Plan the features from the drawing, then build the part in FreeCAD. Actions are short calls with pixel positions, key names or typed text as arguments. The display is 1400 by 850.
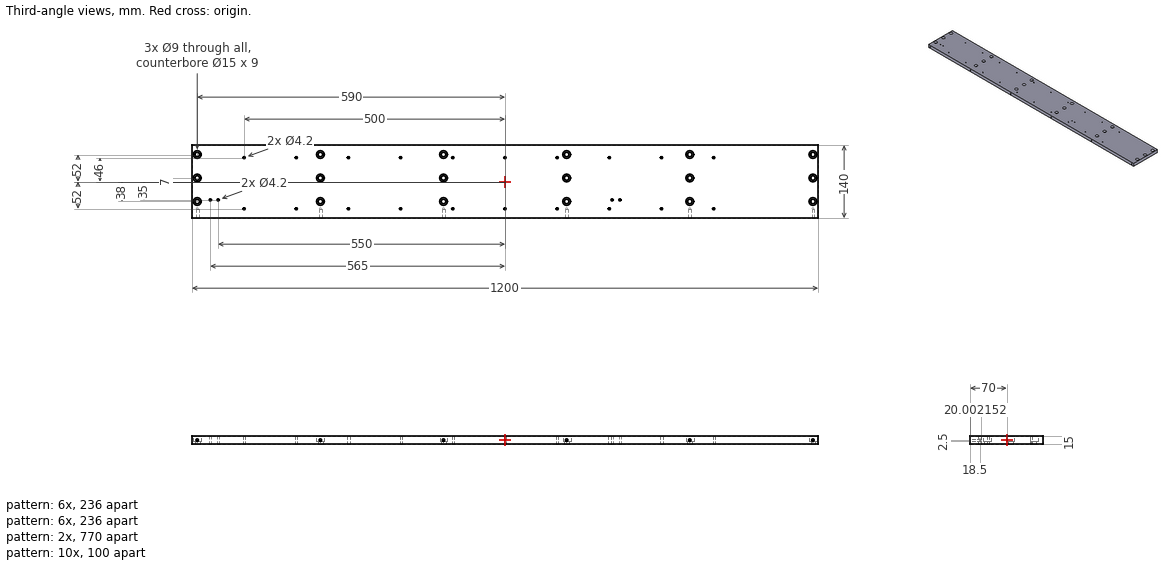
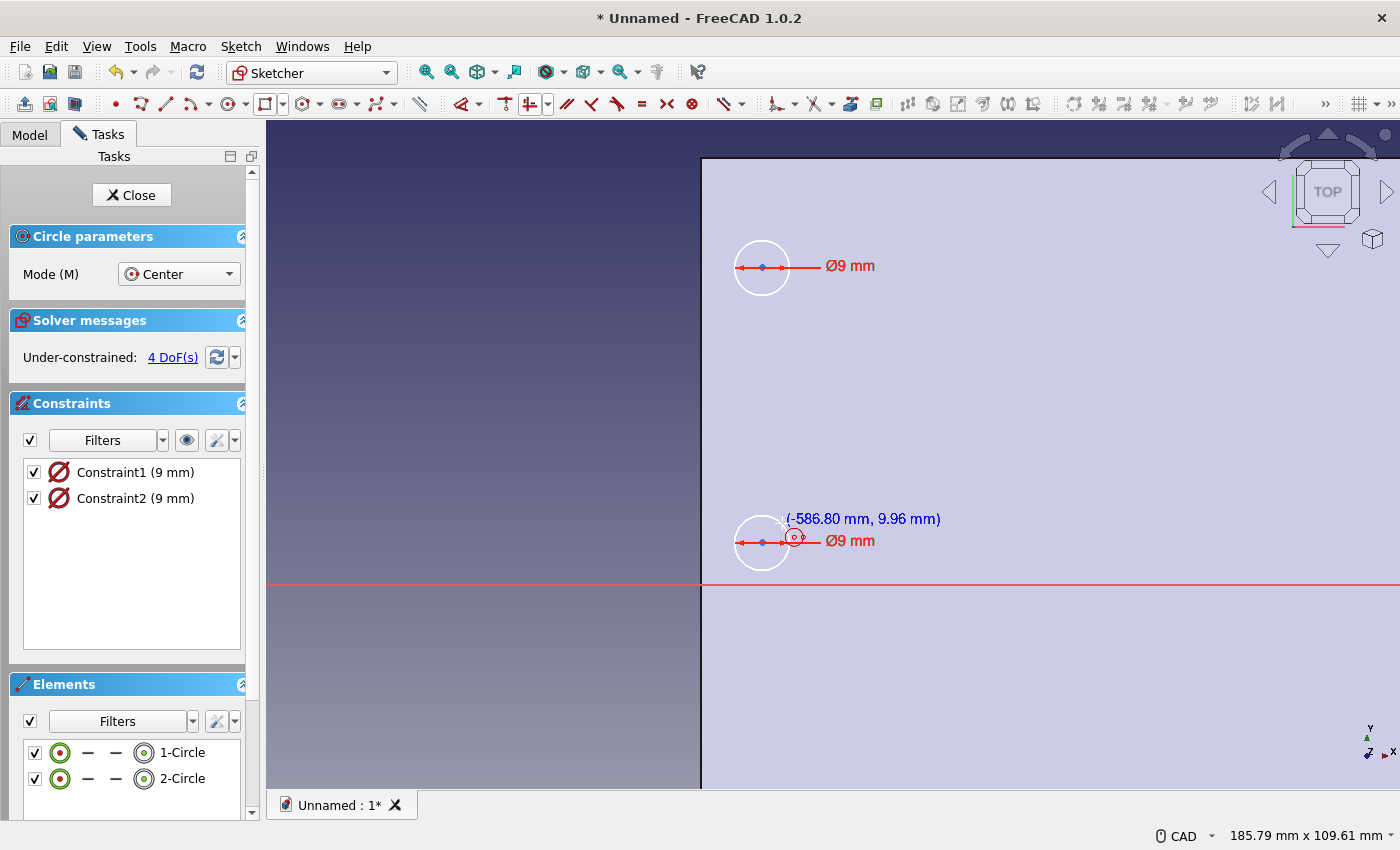
scroll(769, 276, down, 2)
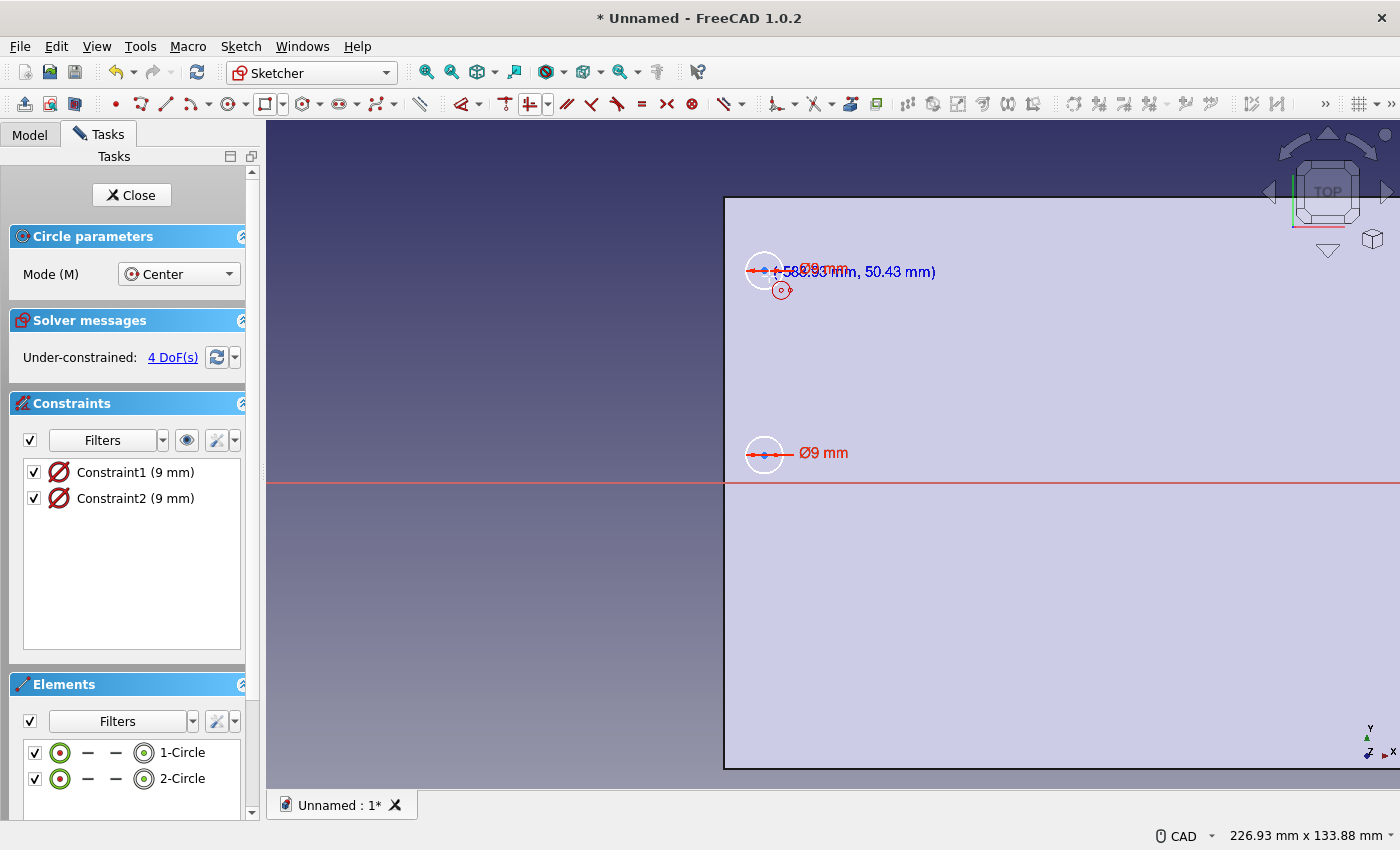
scroll(765, 639, up, 2)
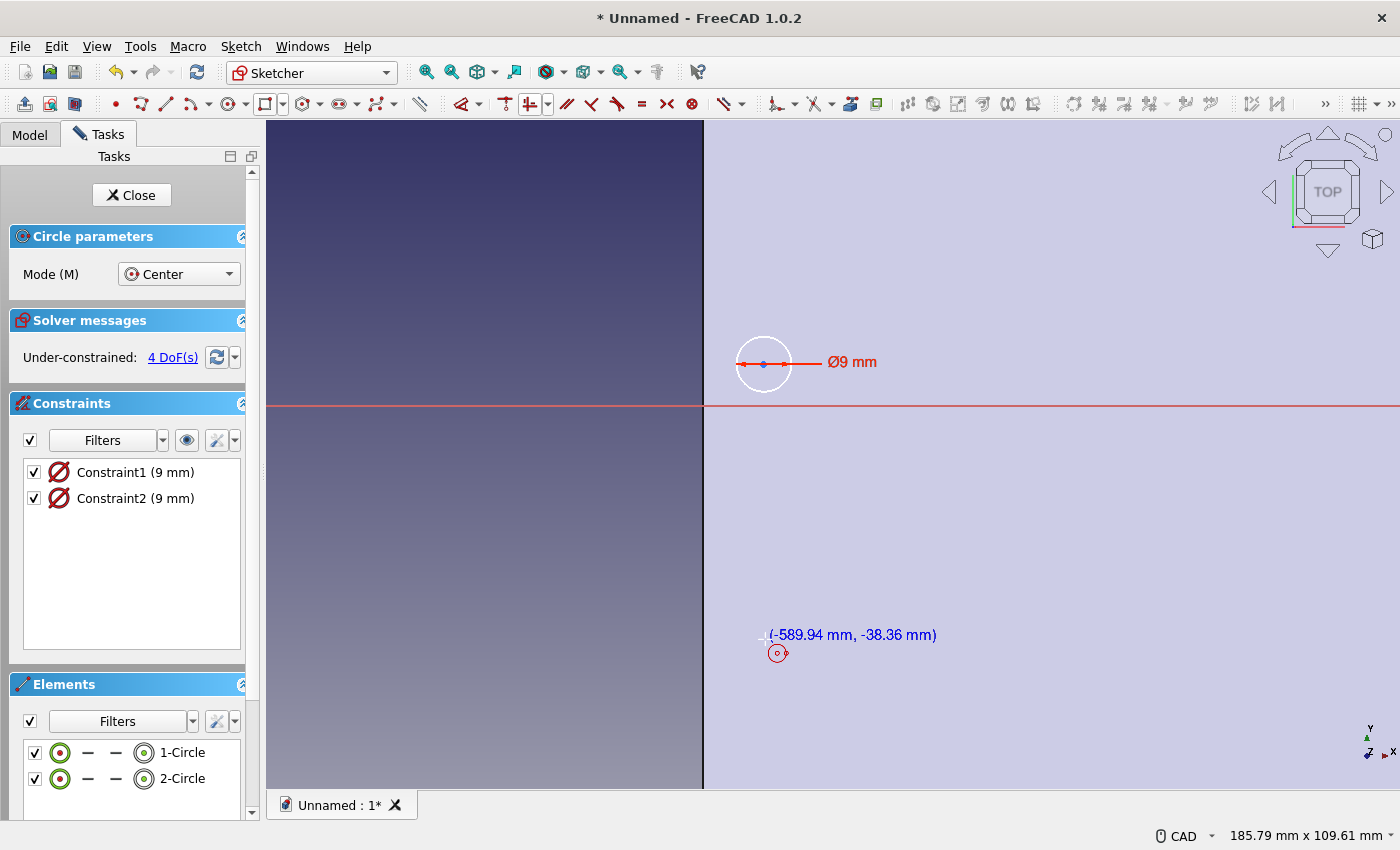
click(764, 638)
move(784, 619)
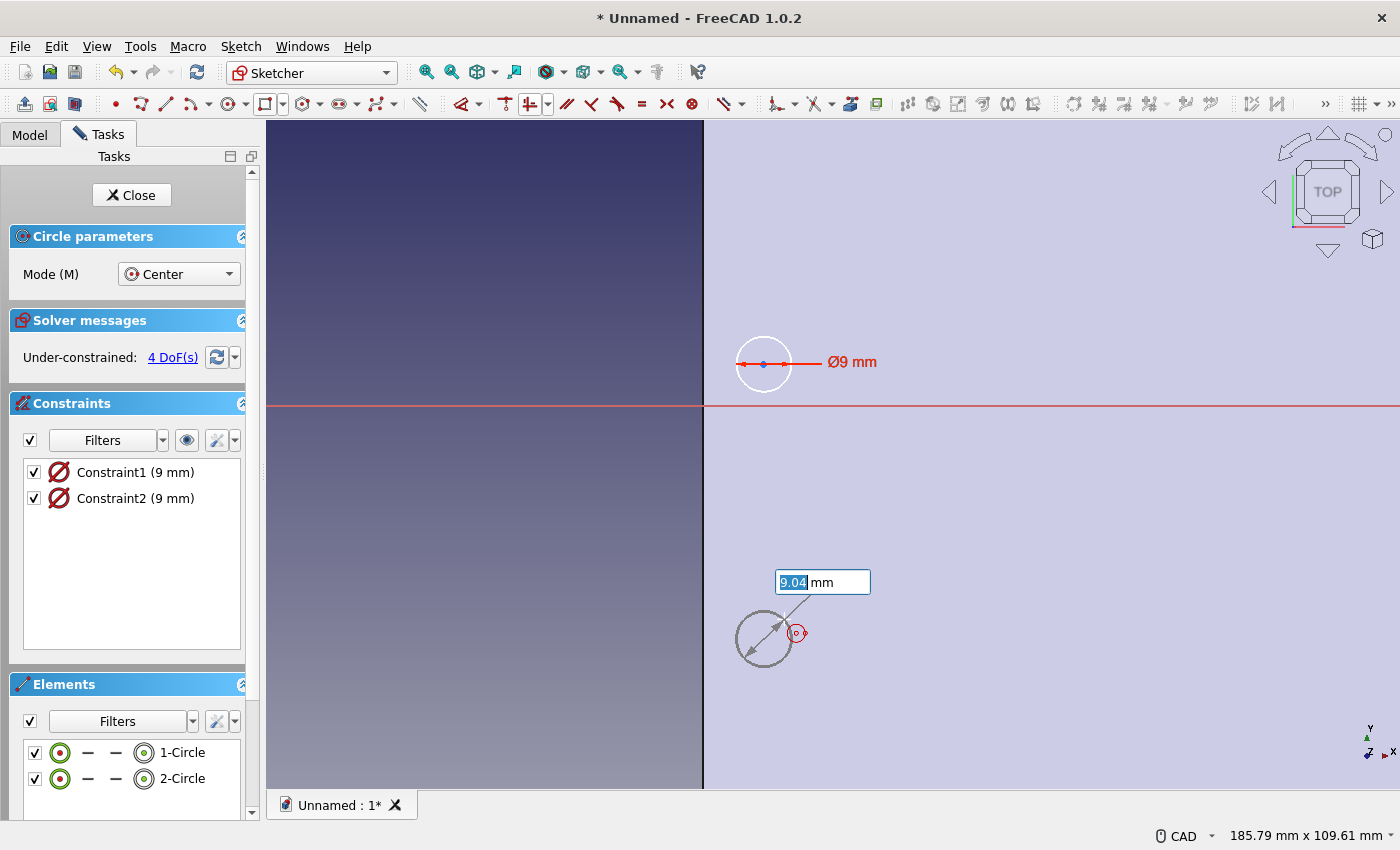
text(9)
key(Return)
key(Escape)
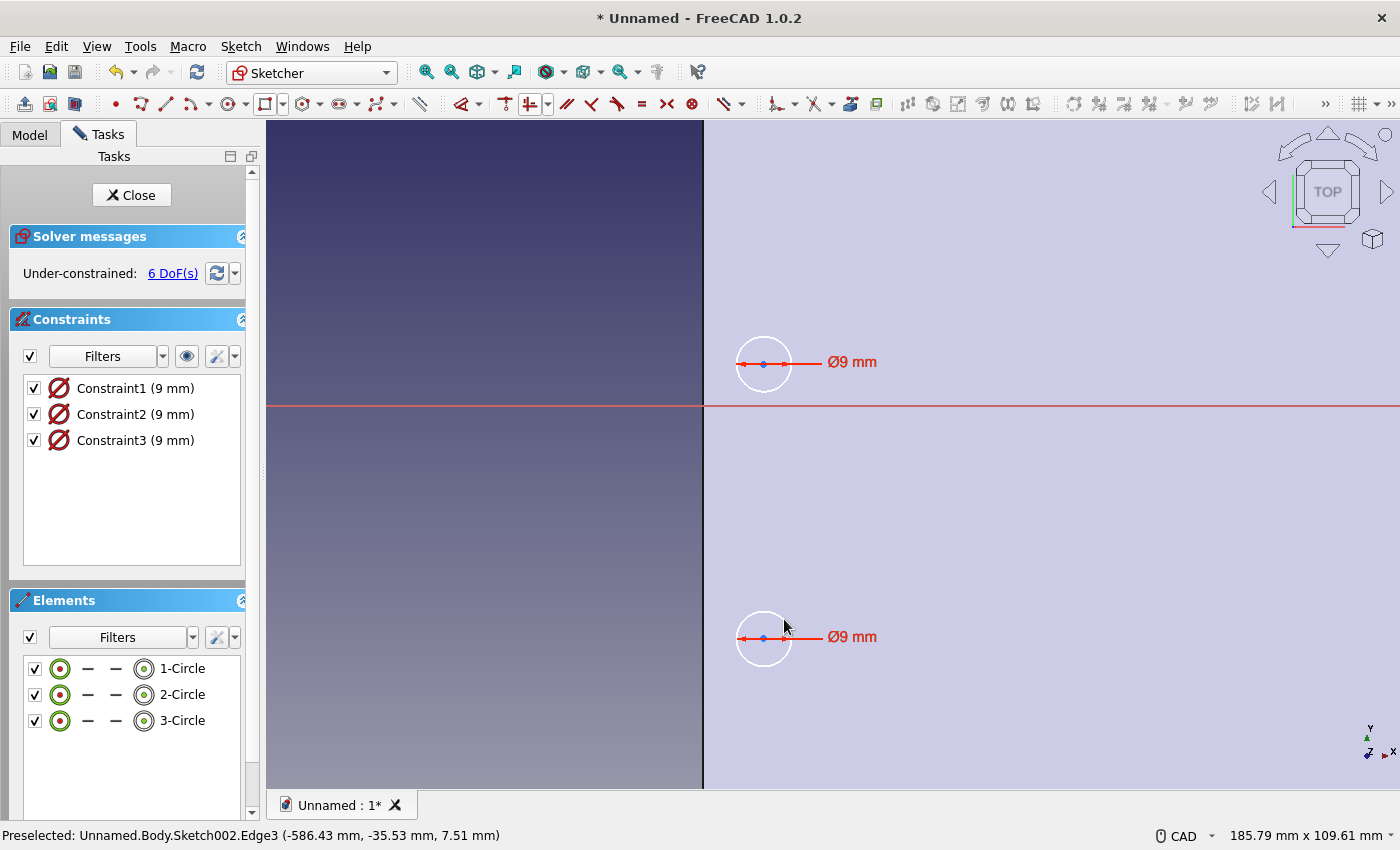
scroll(765, 640, down, 2)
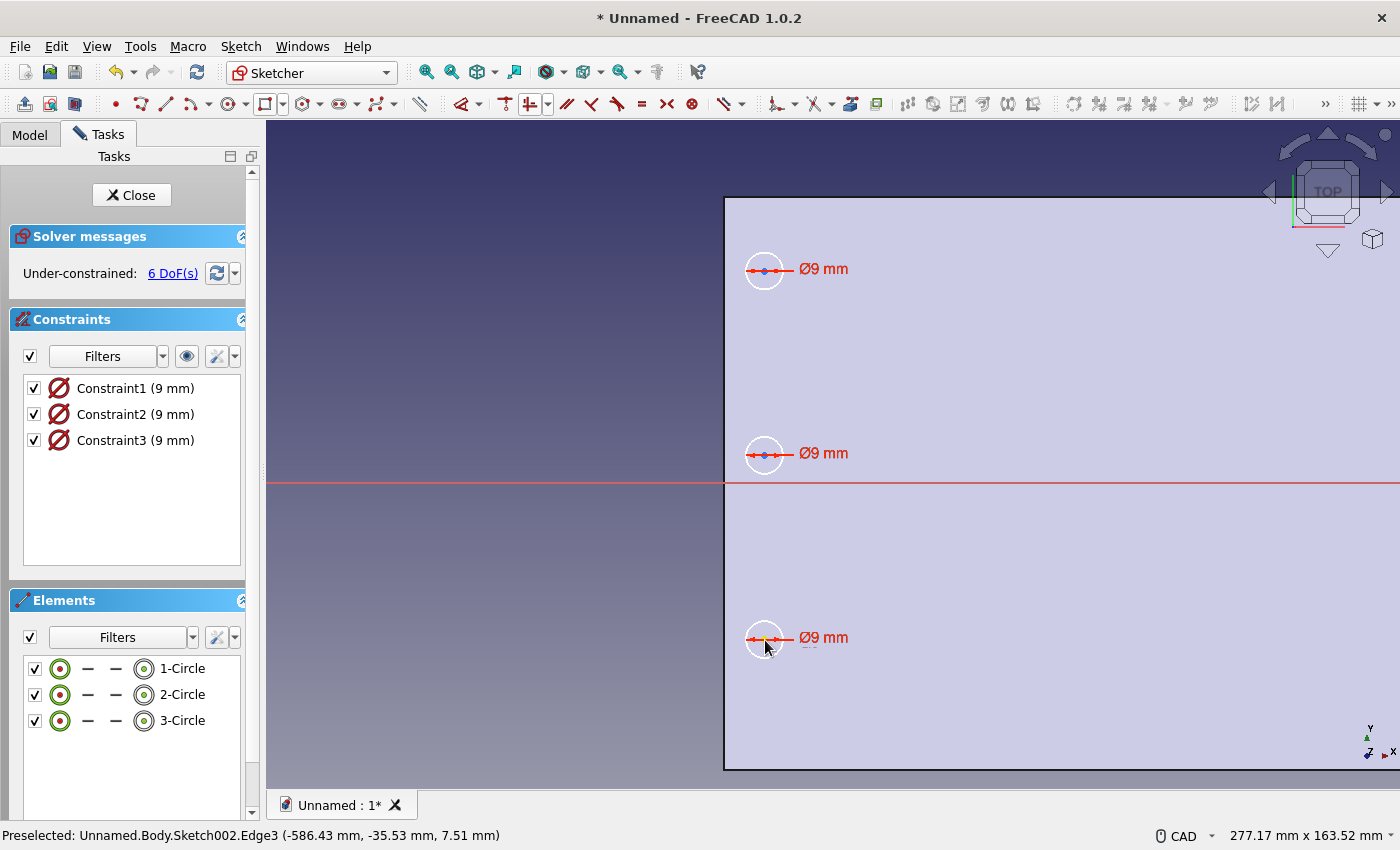
click(764, 271)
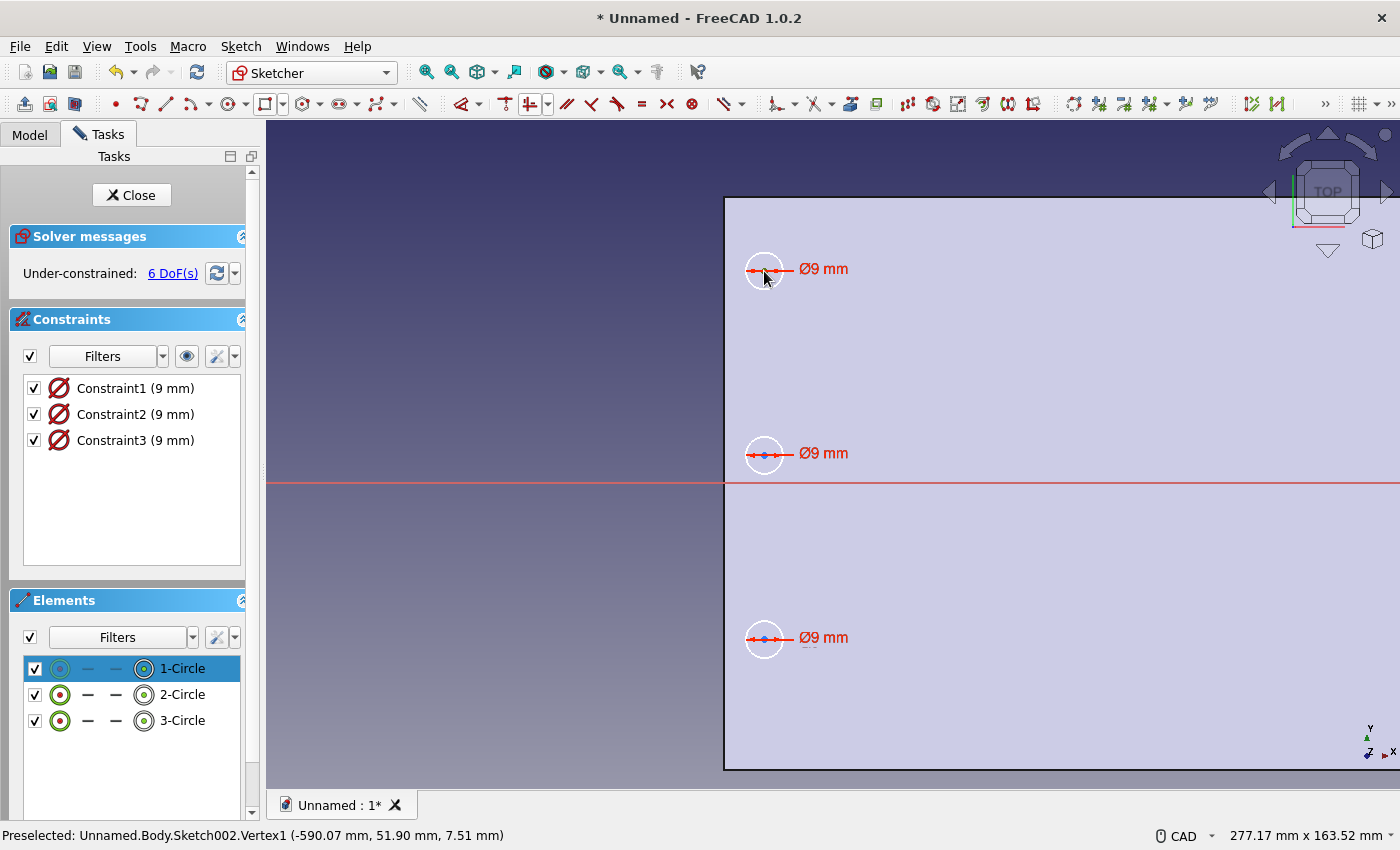
click(764, 455)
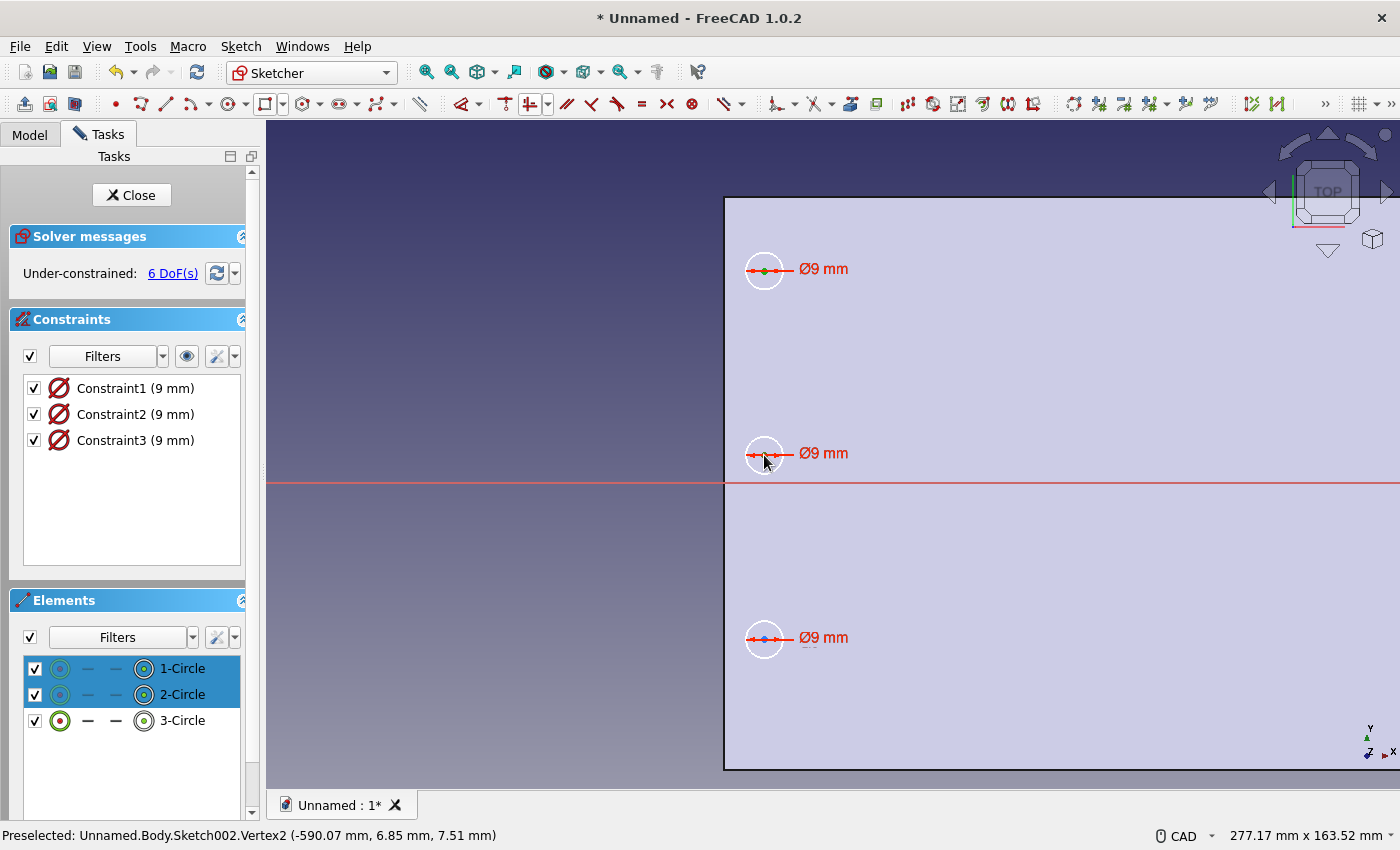
click(548, 104)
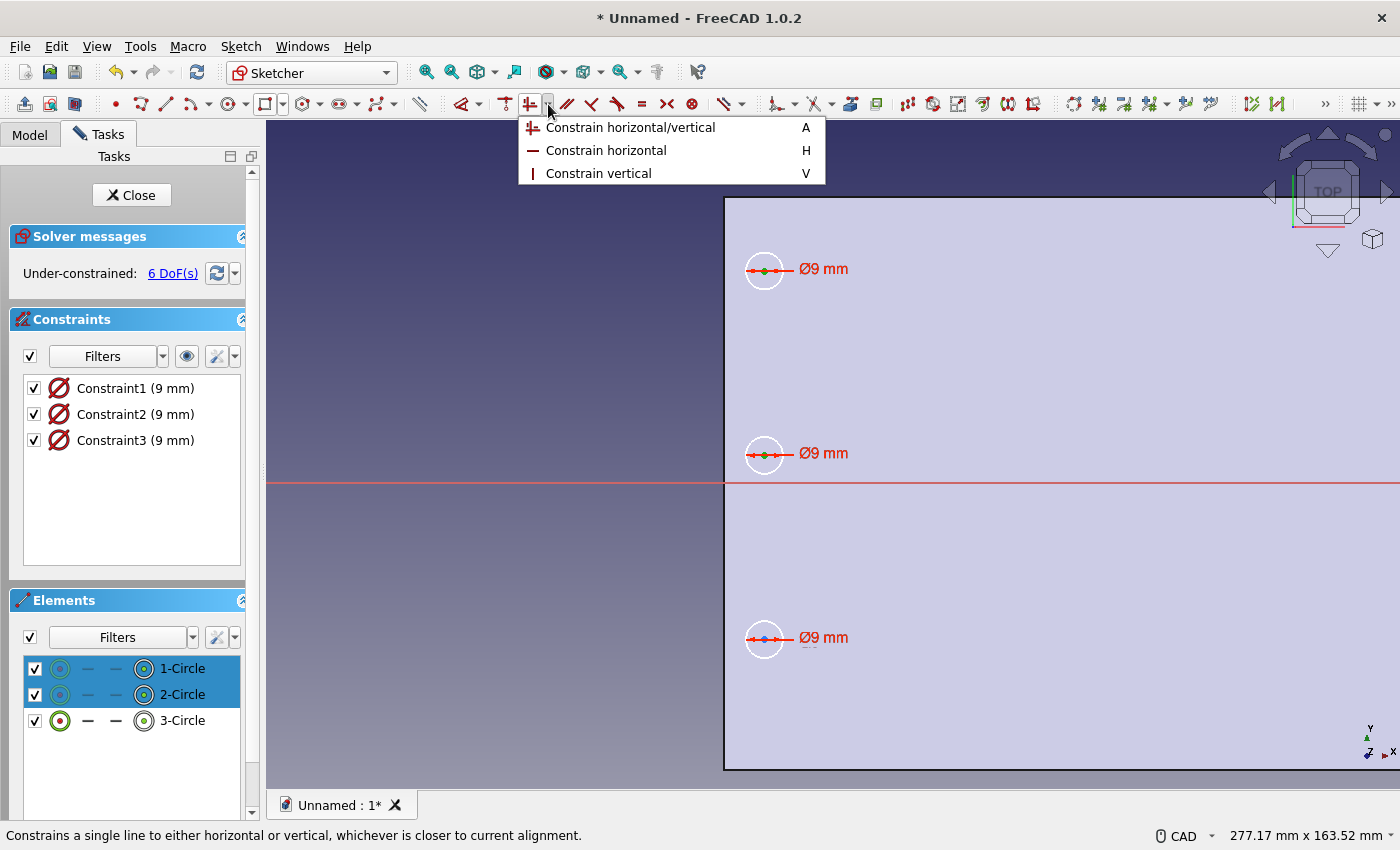
click(672, 174)